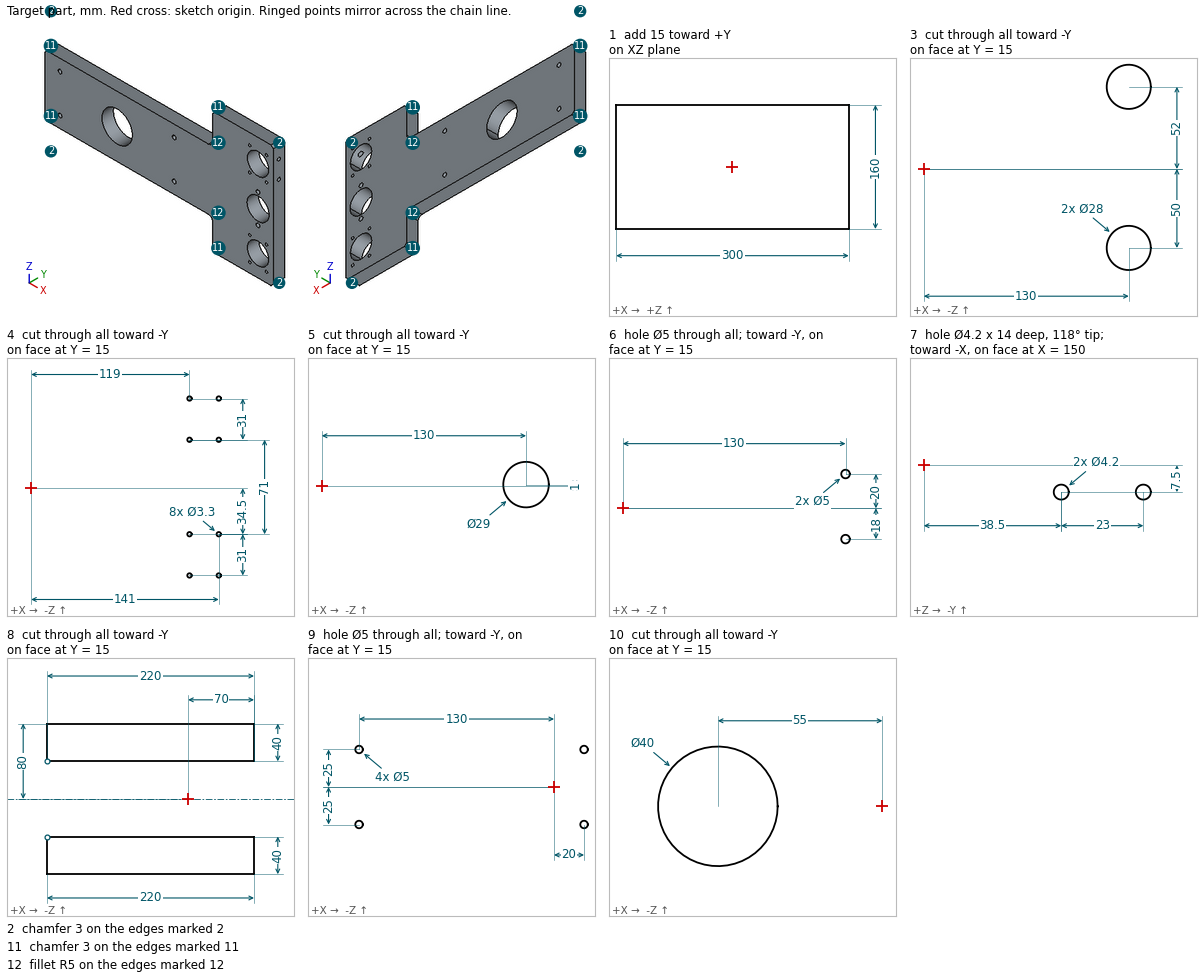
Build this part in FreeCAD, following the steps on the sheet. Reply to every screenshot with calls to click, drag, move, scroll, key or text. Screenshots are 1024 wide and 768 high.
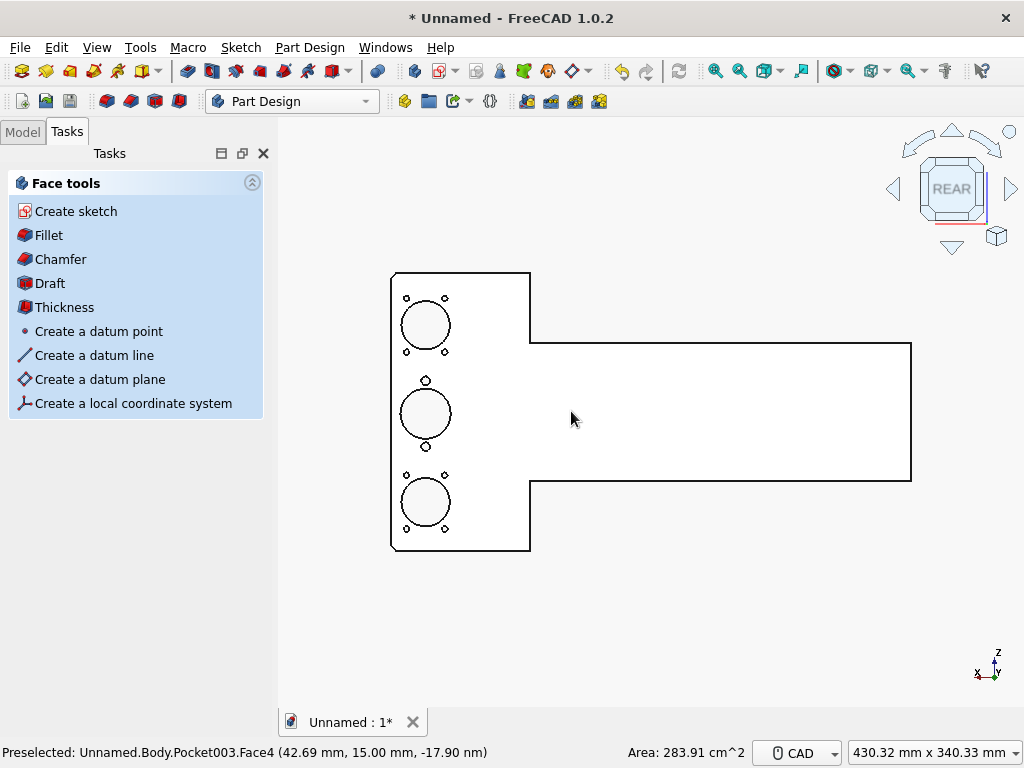
click(440, 72)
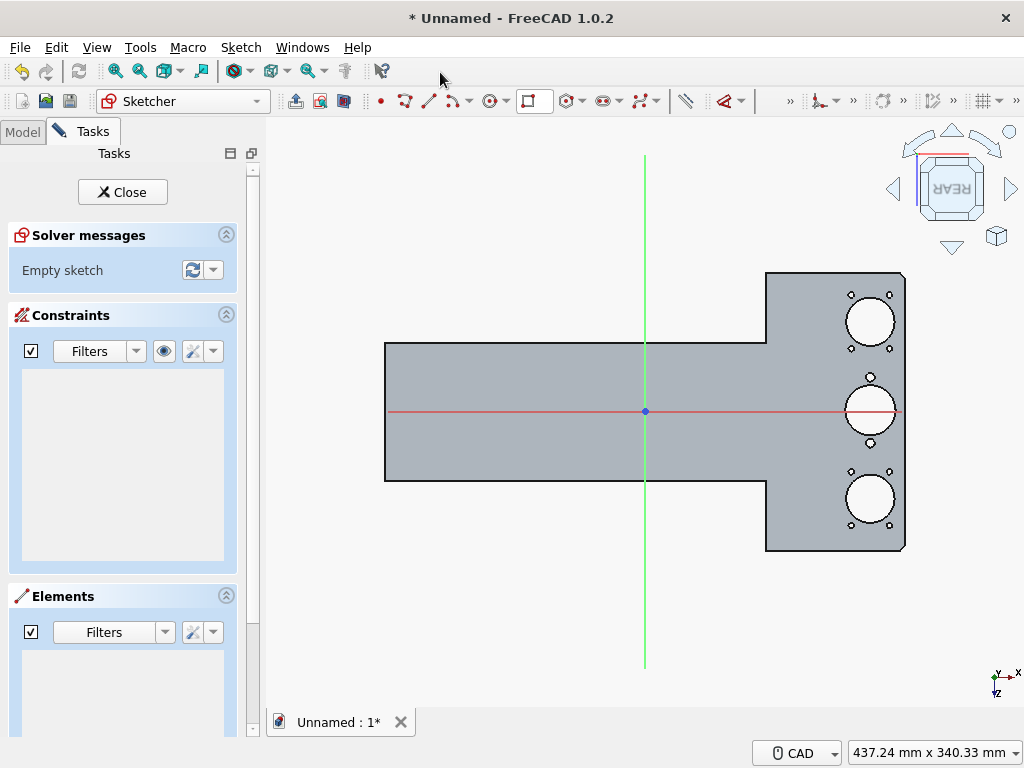
scroll(495, 412, up, 2)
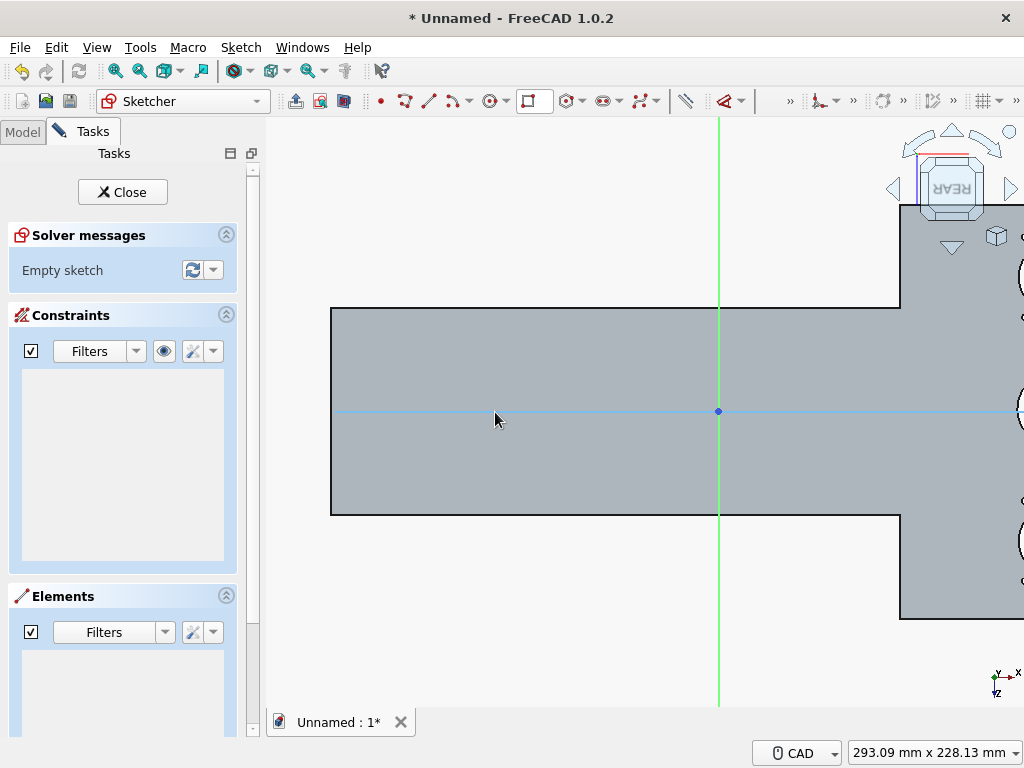
click(490, 102)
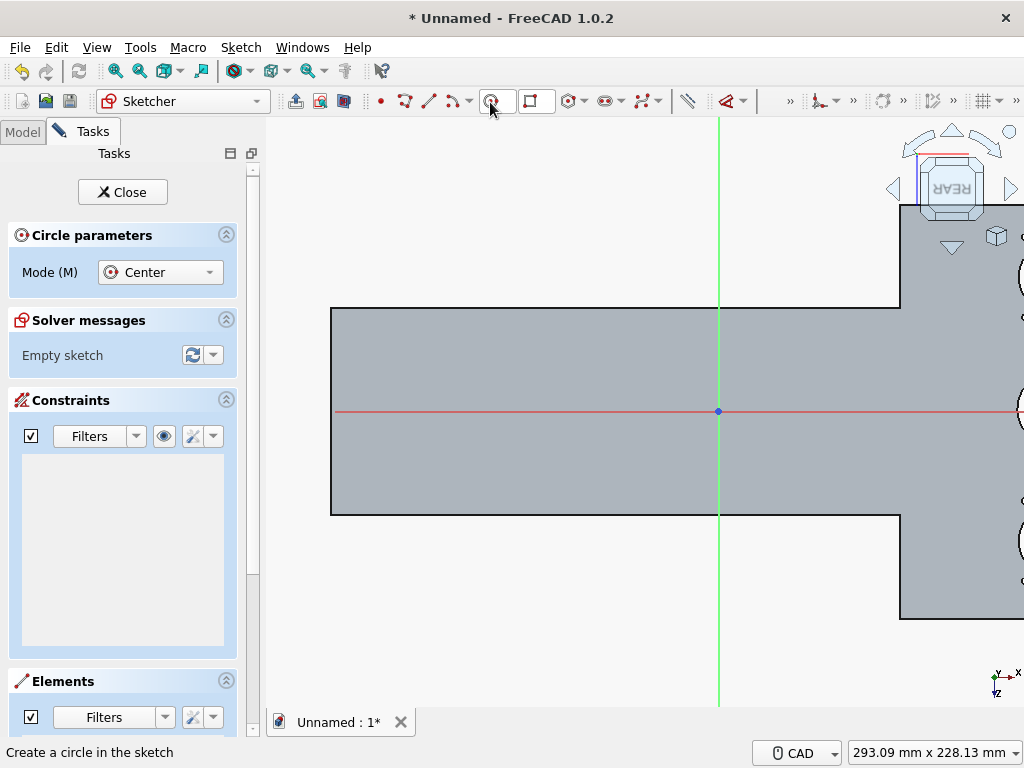
scroll(382, 347, up, 7)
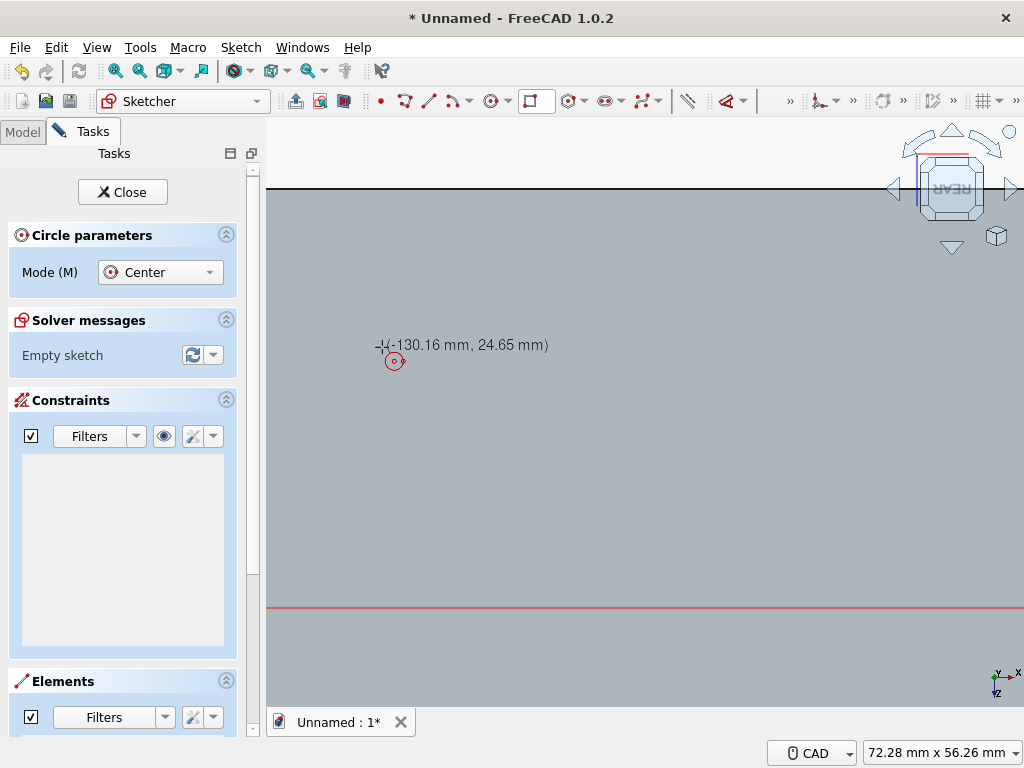
scroll(382, 348, down, 7)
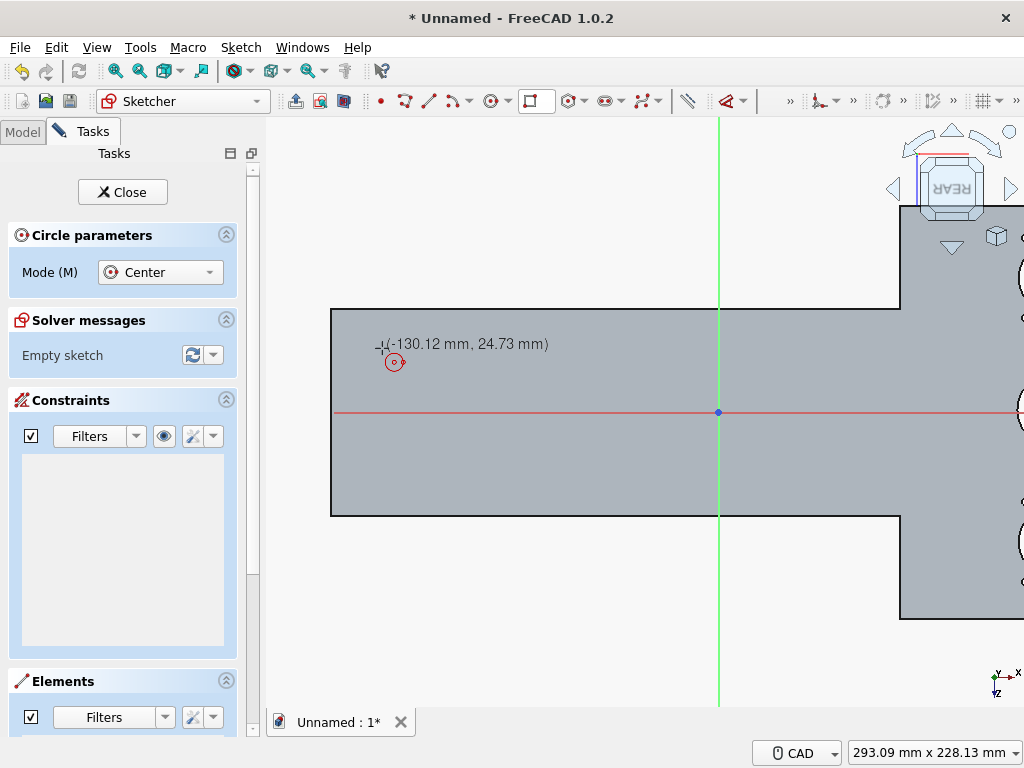
click(382, 348)
move(387, 343)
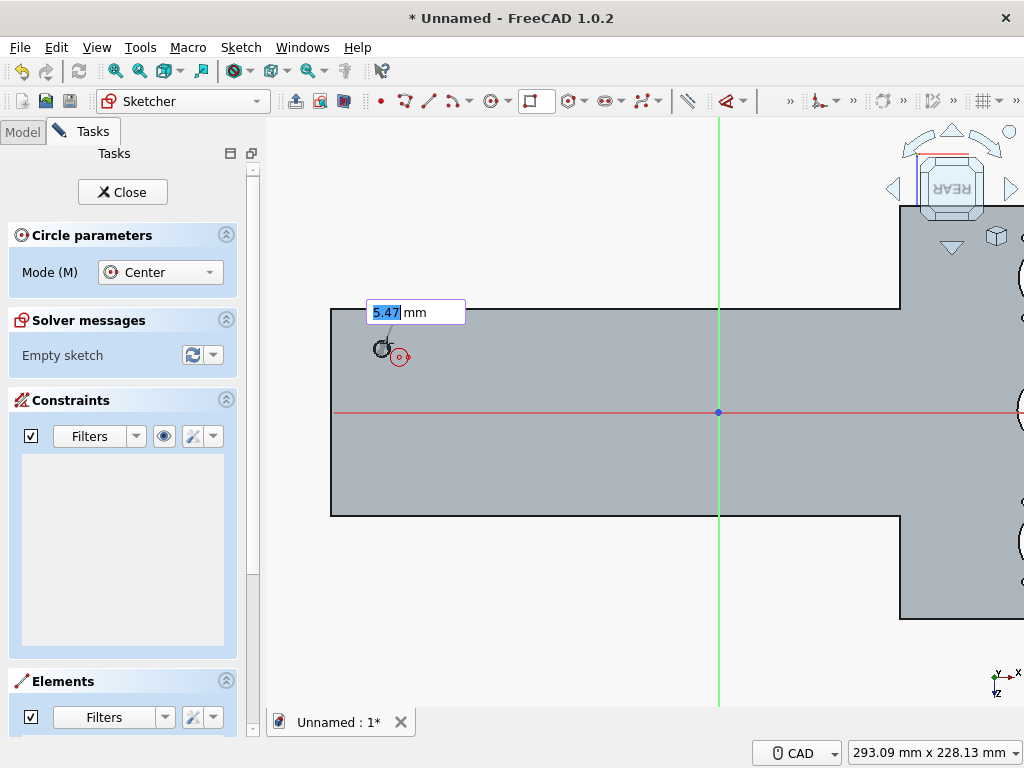
text(5)
key(Return)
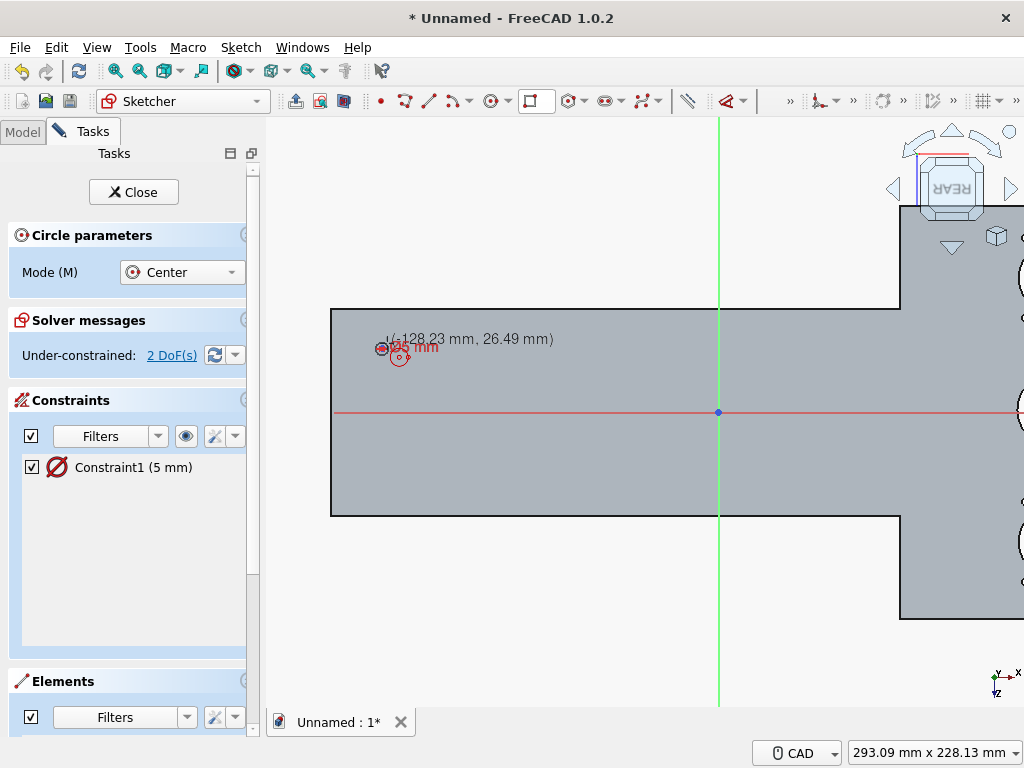
scroll(382, 477, up, 7)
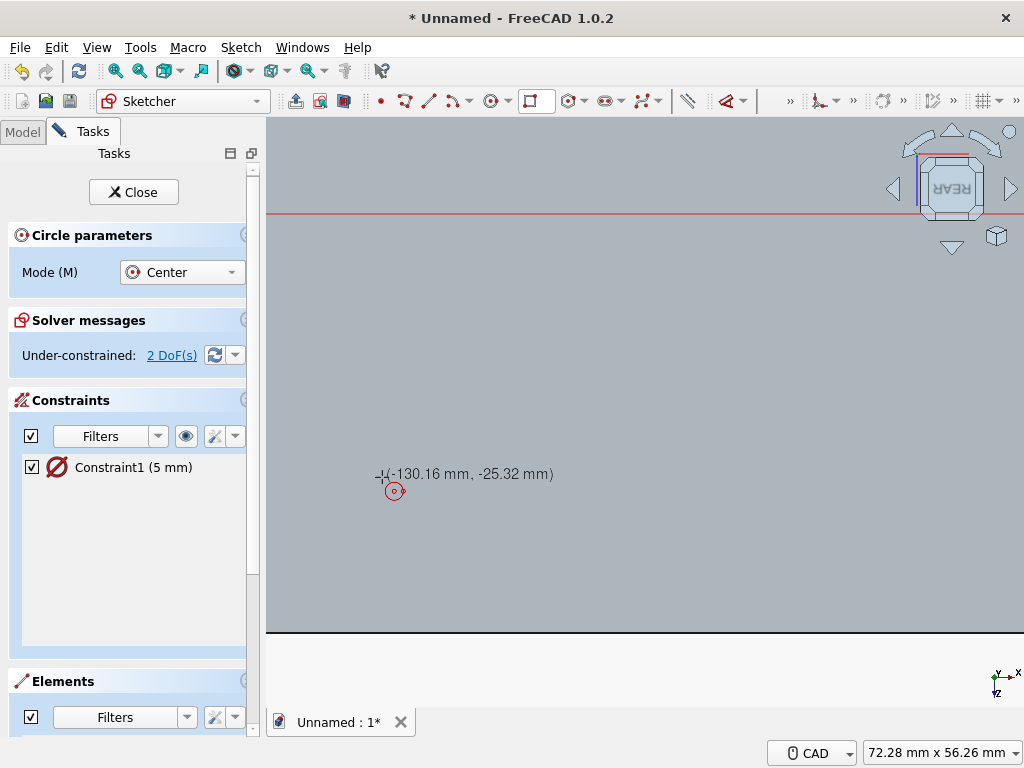
scroll(382, 477, down, 7)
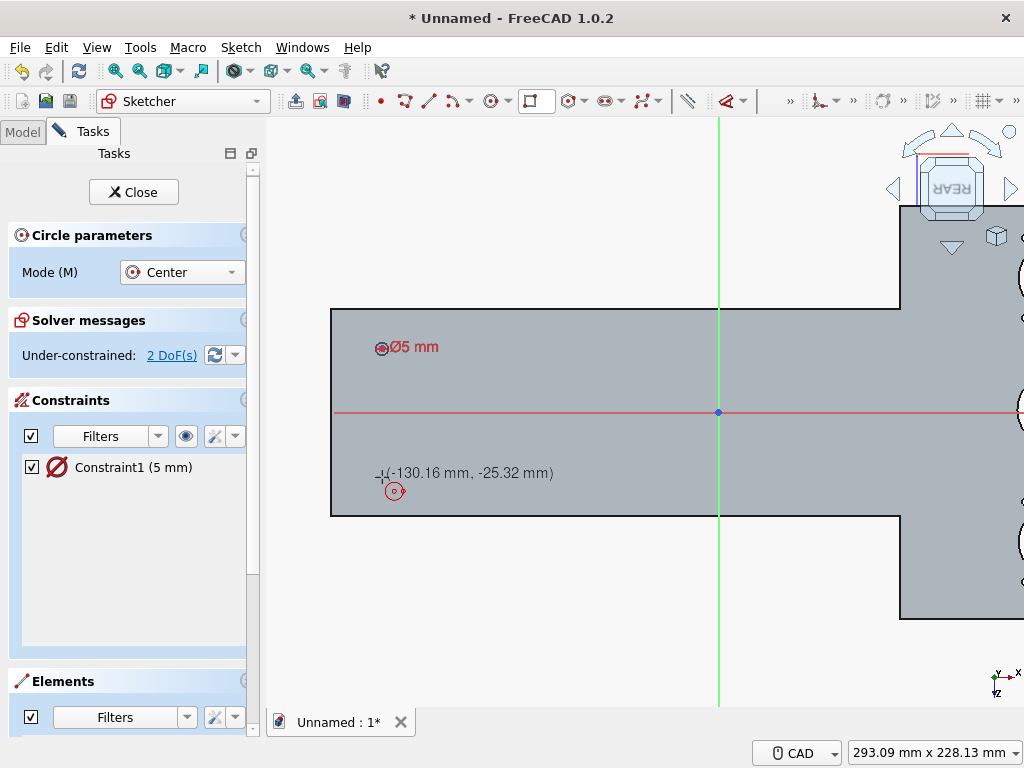
click(382, 477)
move(387, 473)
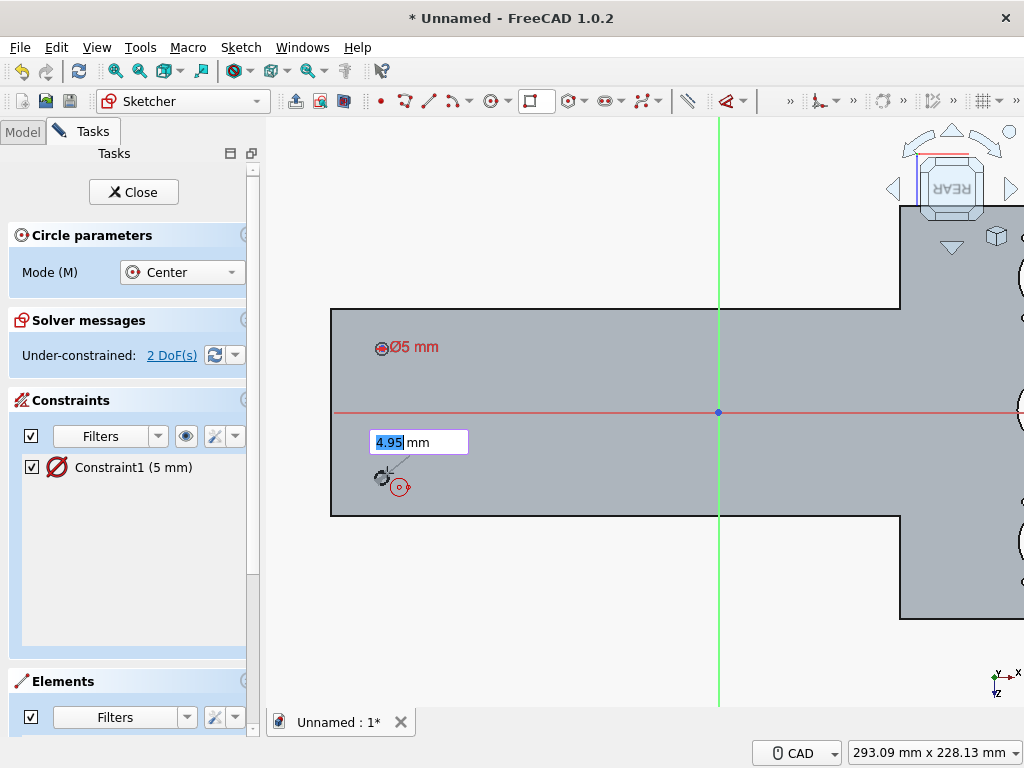
text(5)
key(Return)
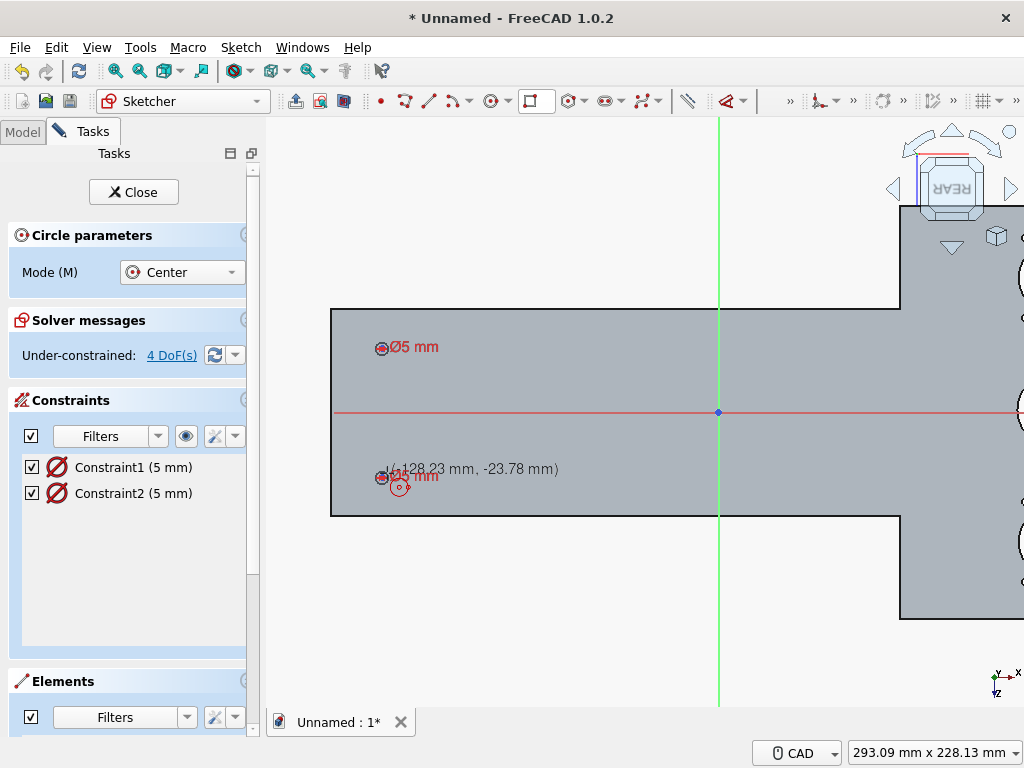
scroll(770, 477, up, 7)